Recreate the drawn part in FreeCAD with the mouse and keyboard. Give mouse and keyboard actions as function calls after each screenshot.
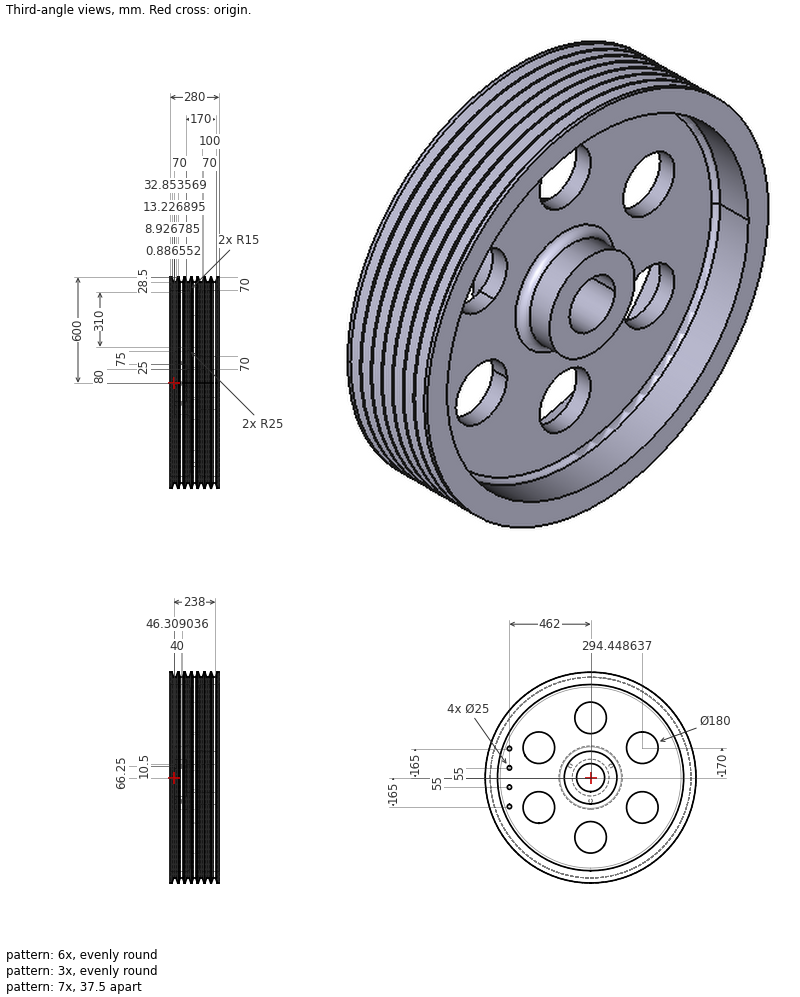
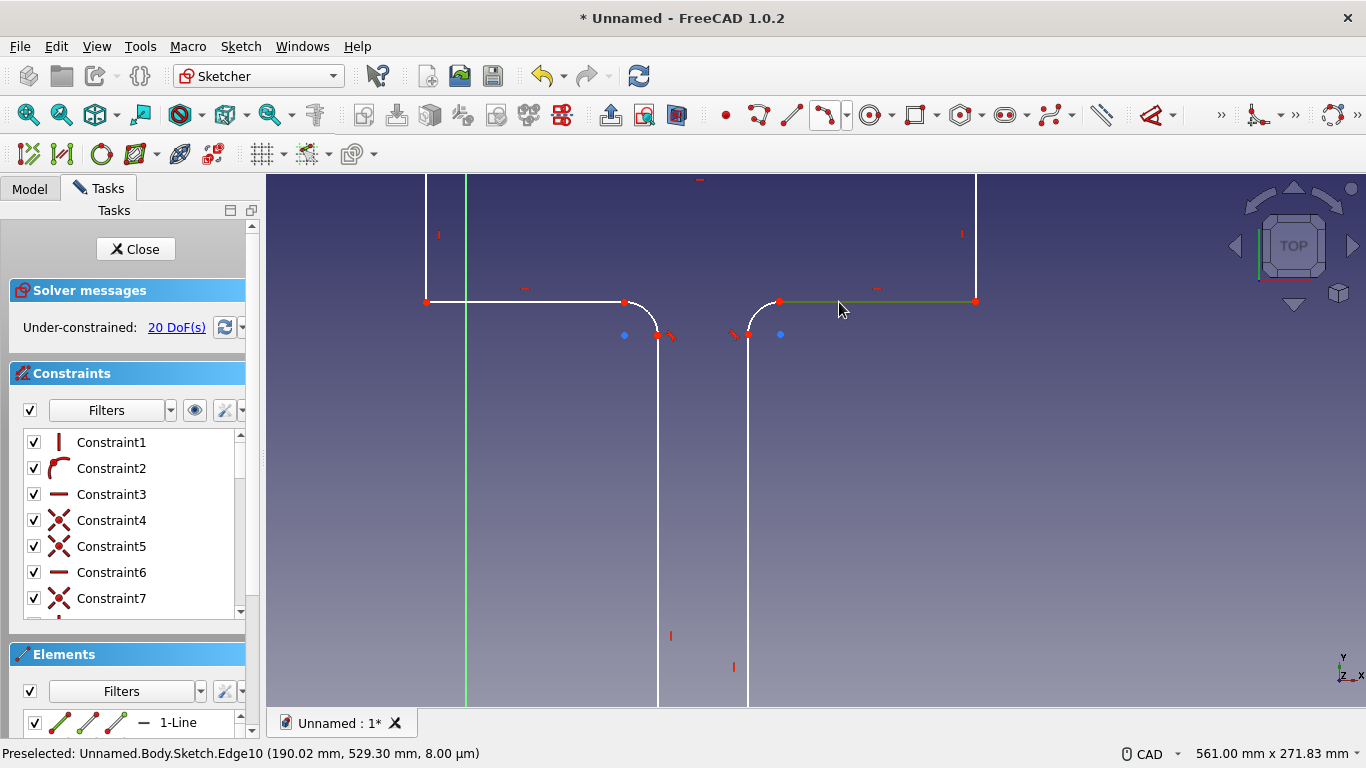
click(765, 306)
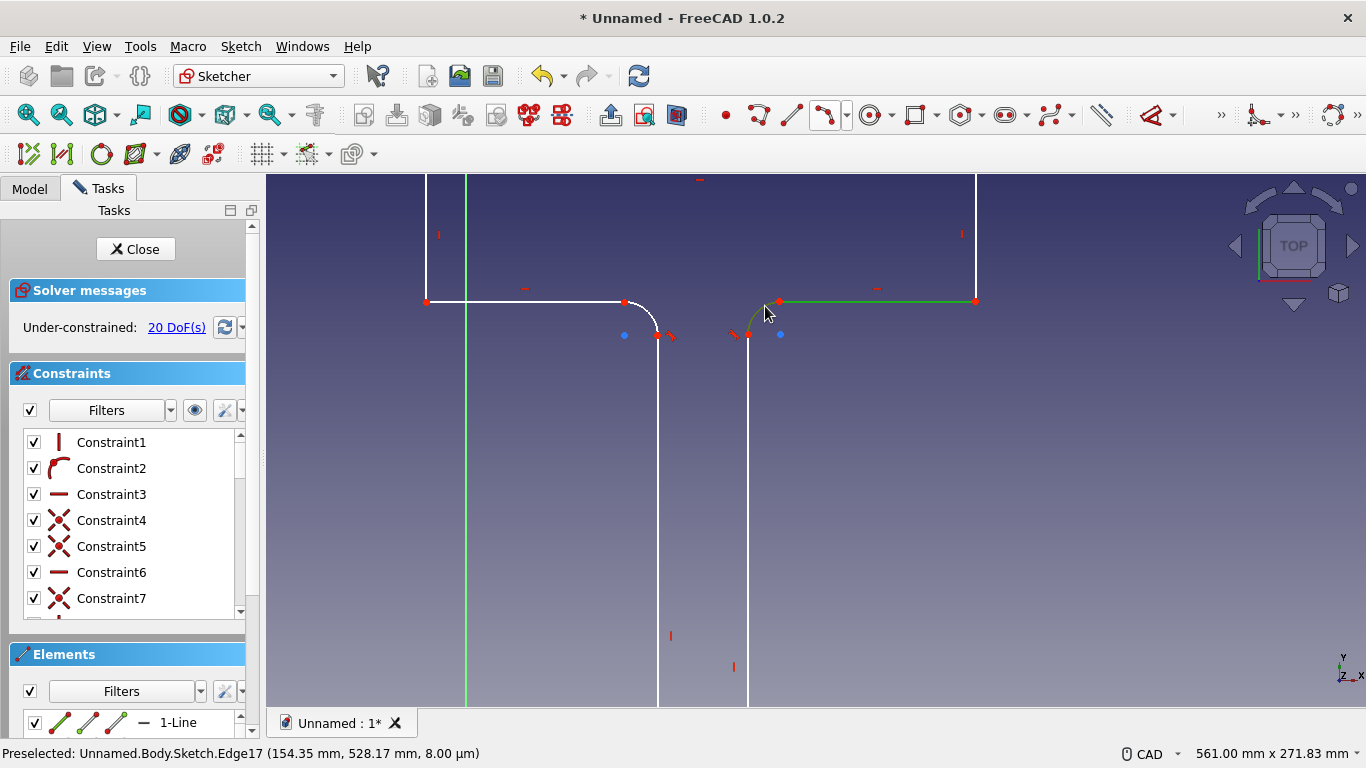
key(t)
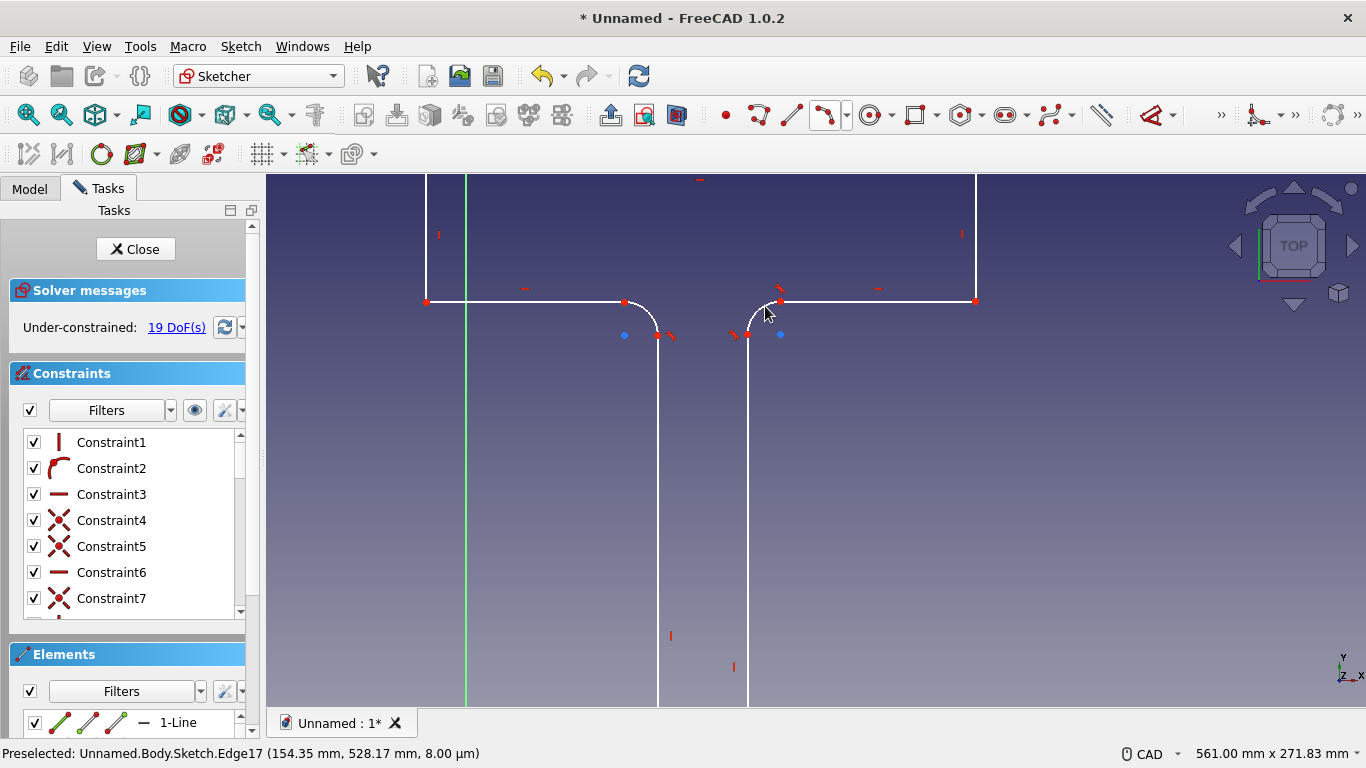
click(486, 302)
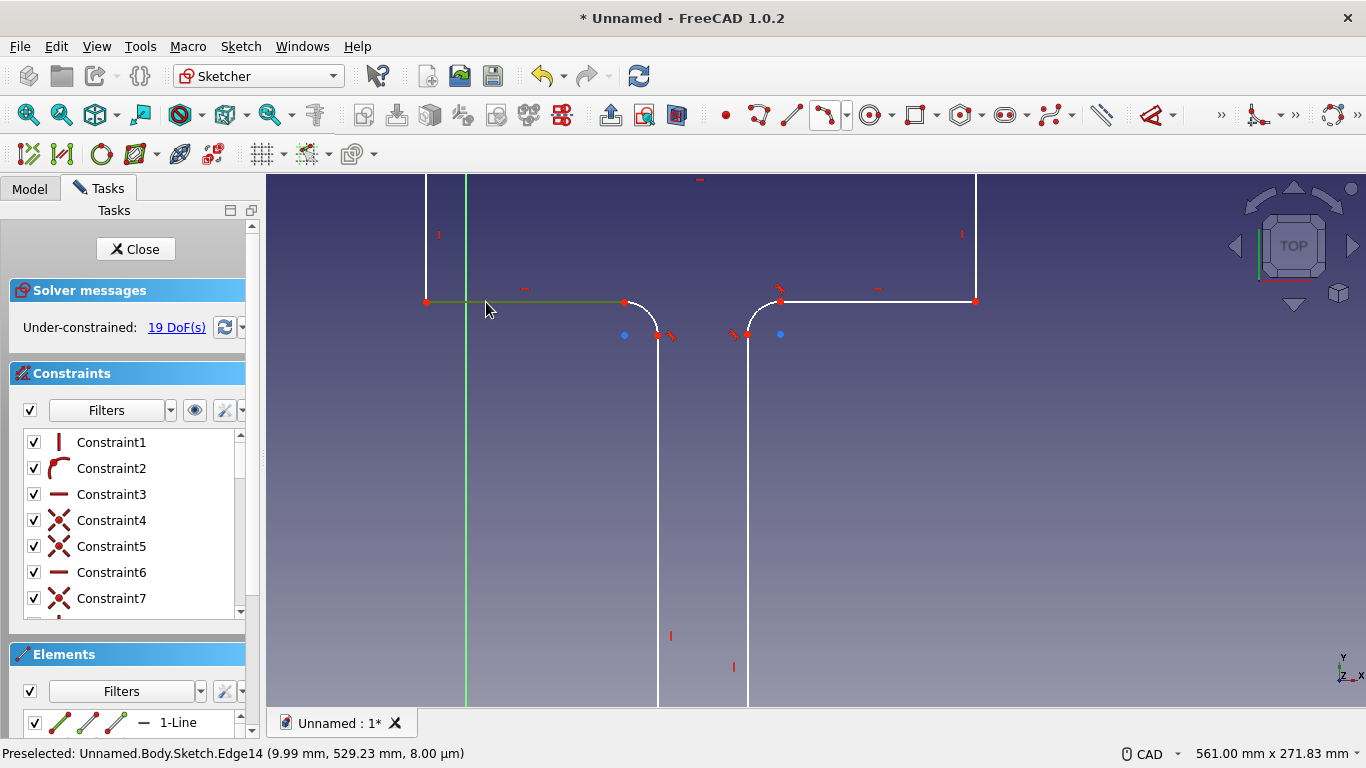
click(654, 321)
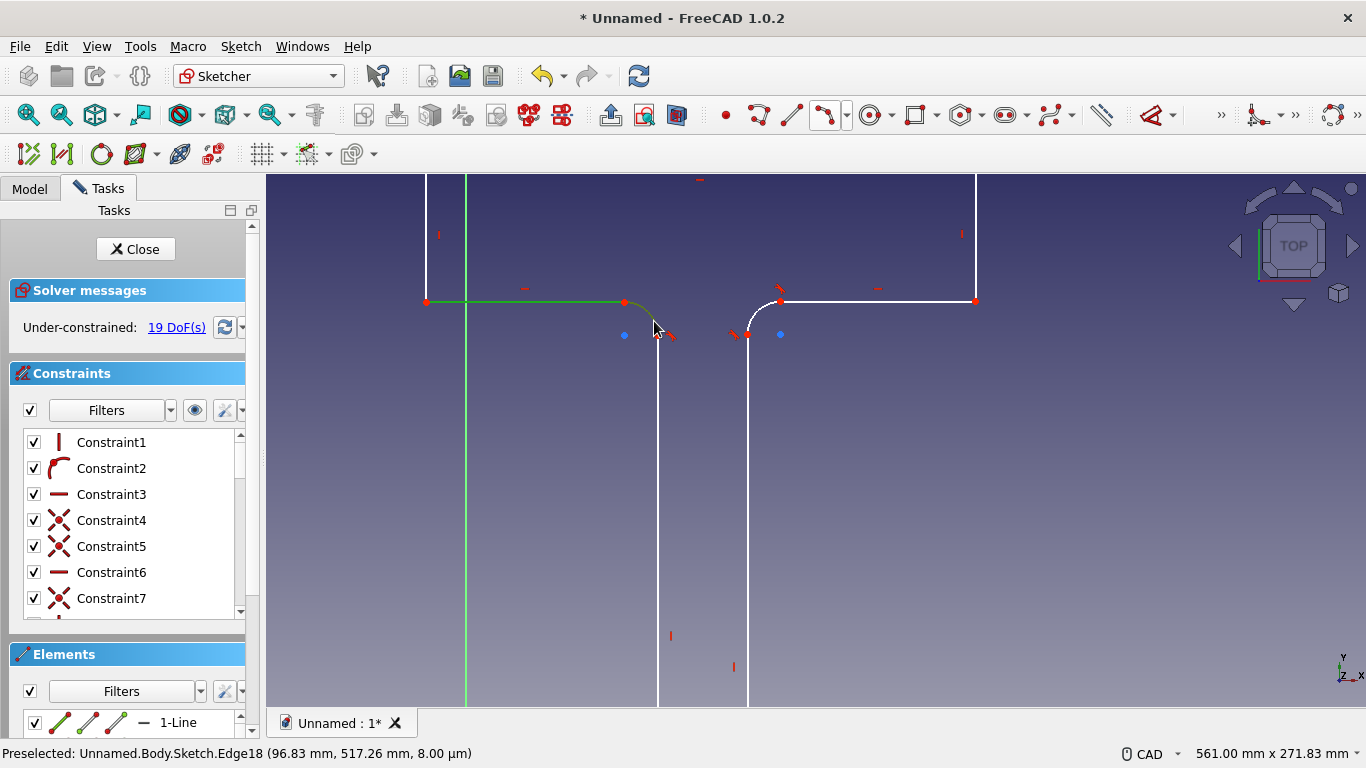
key(t)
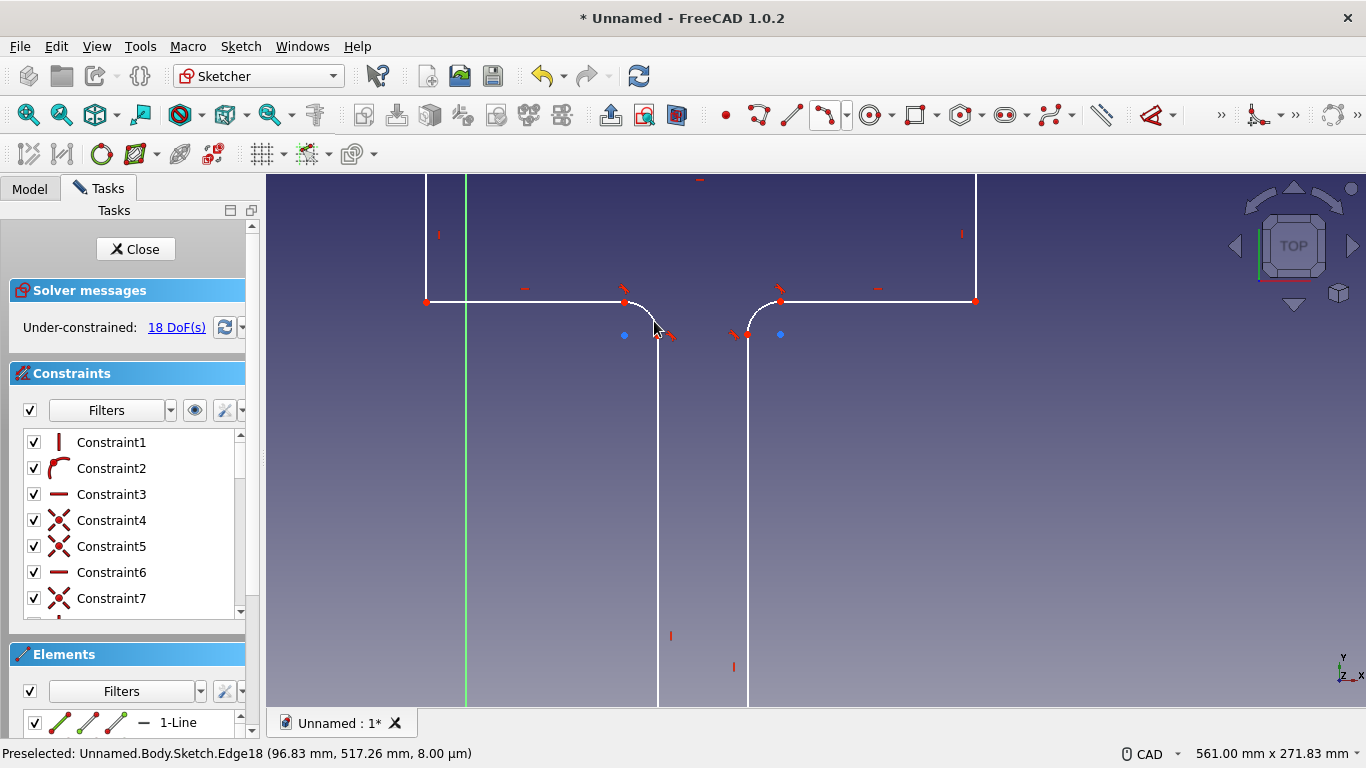
scroll(767, 306, down, 6)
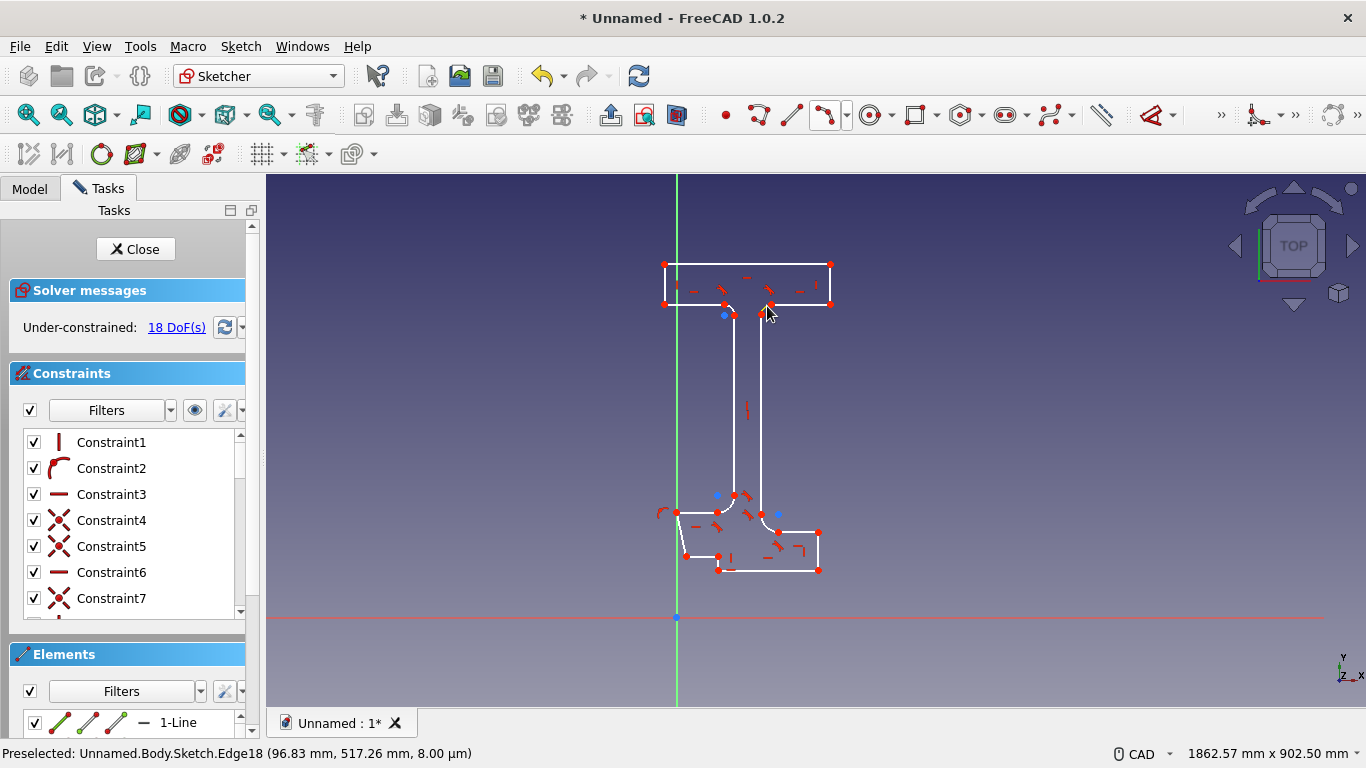
scroll(680, 526, up, 9)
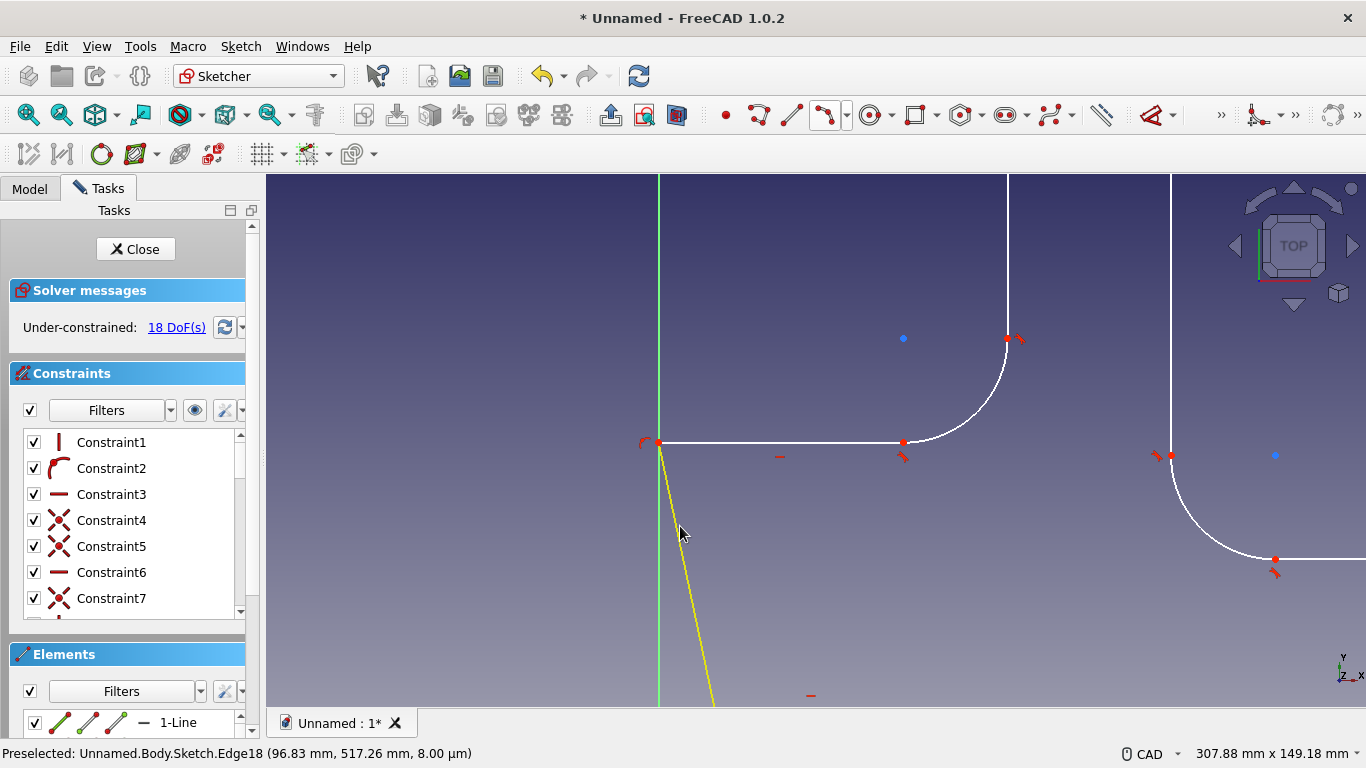
click(675, 523)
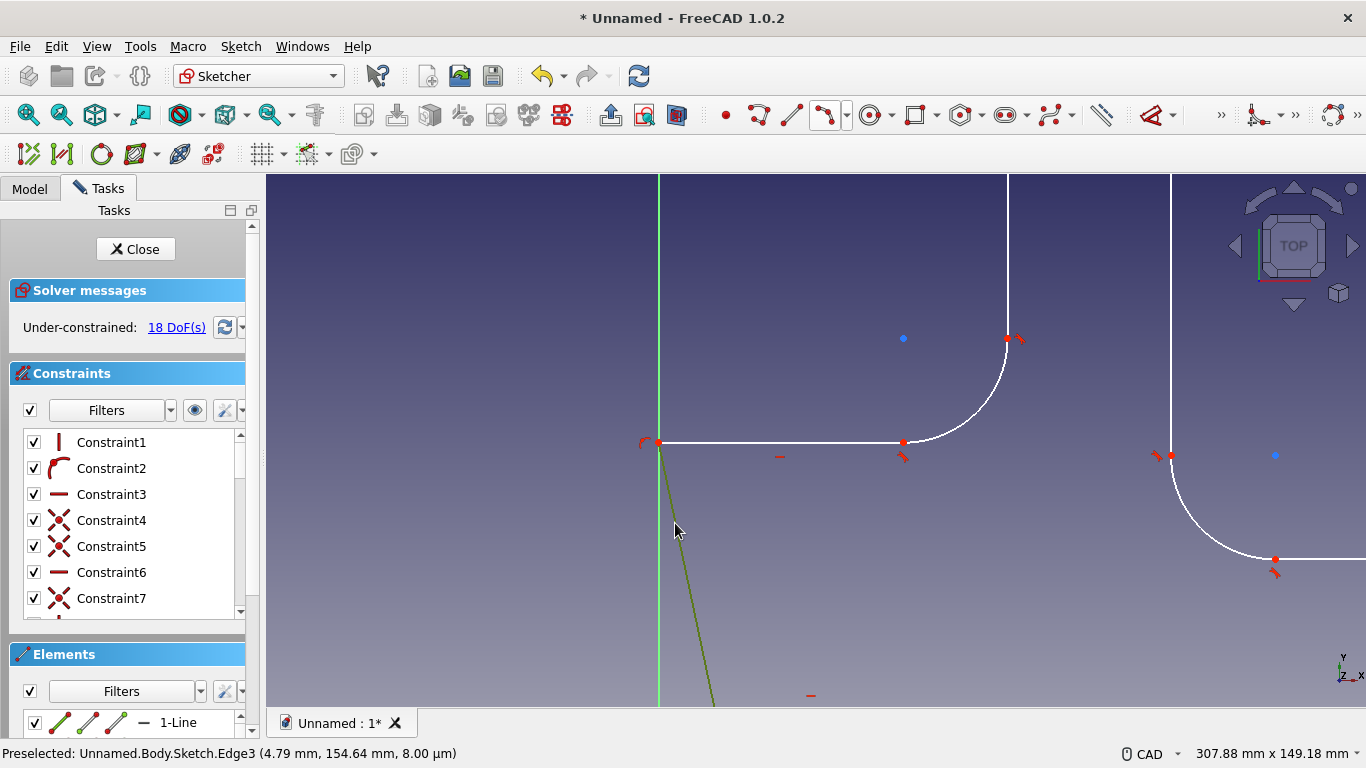
key(v)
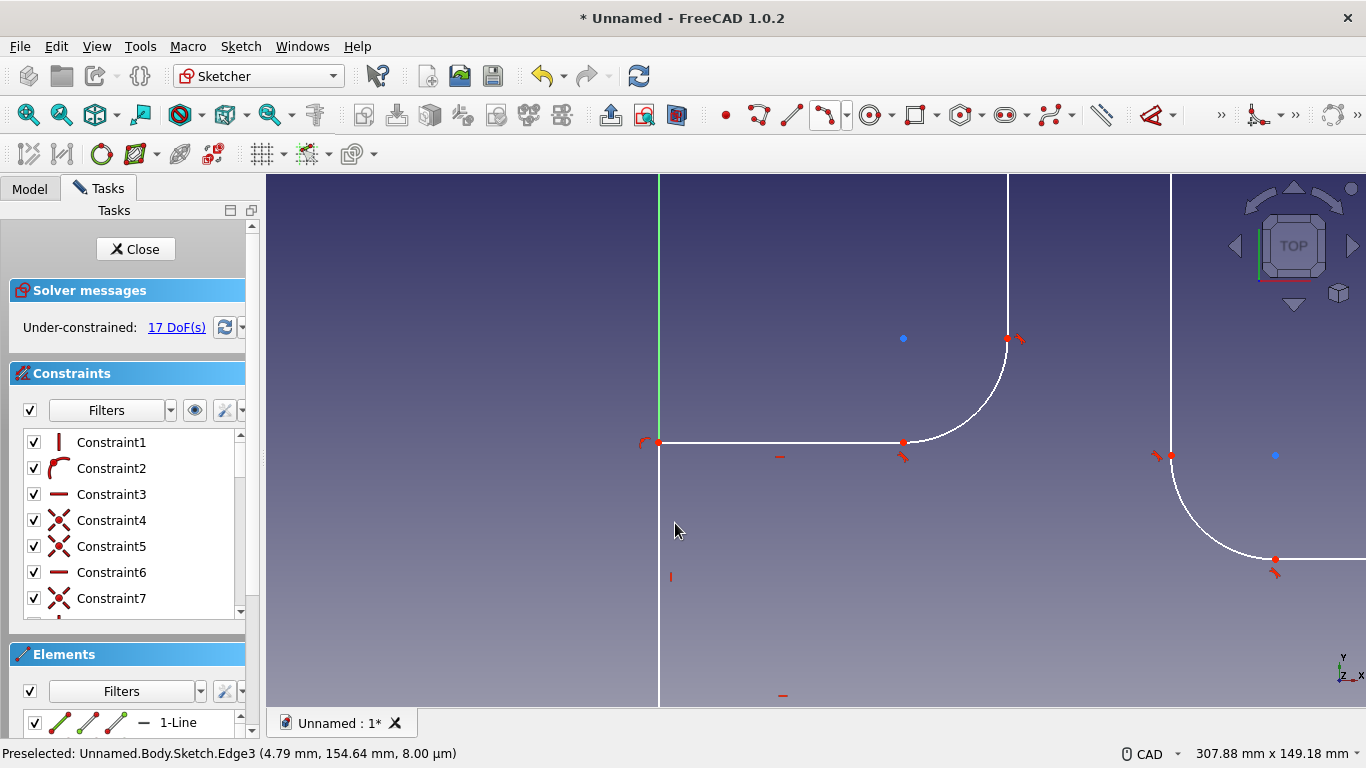
scroll(680, 527, down, 9)